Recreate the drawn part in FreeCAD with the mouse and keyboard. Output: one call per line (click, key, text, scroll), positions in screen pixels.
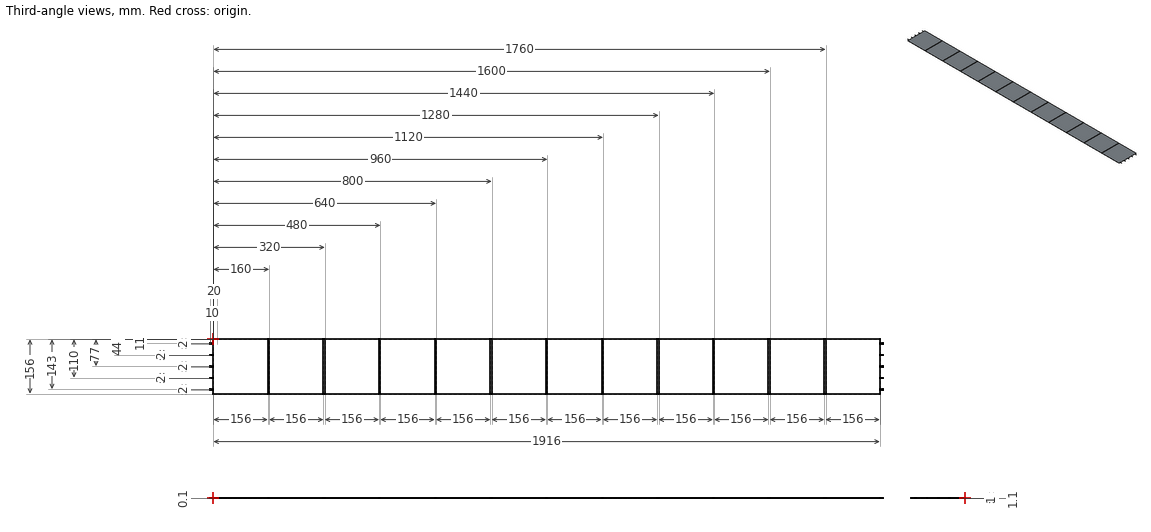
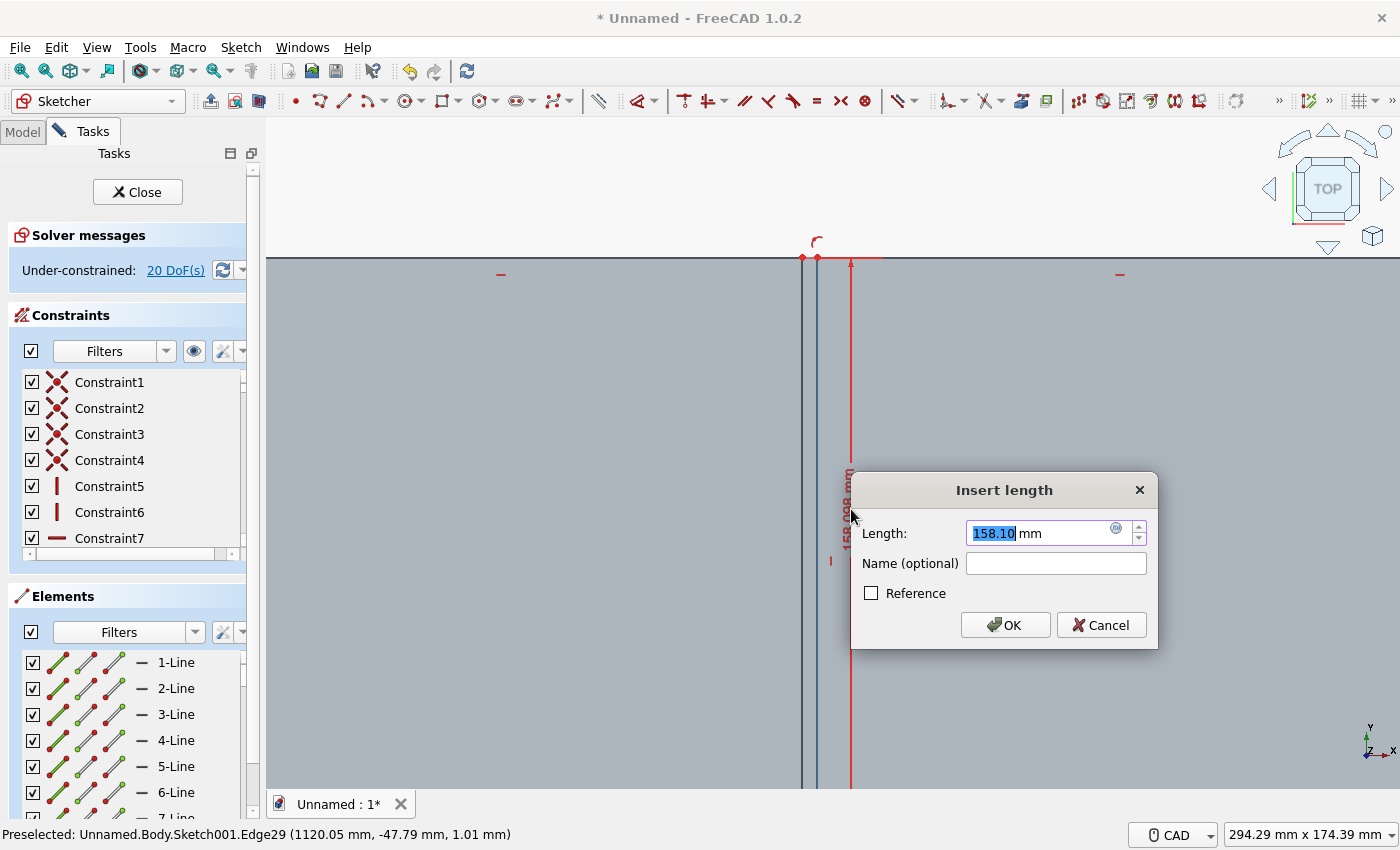
text(156)
key(Return)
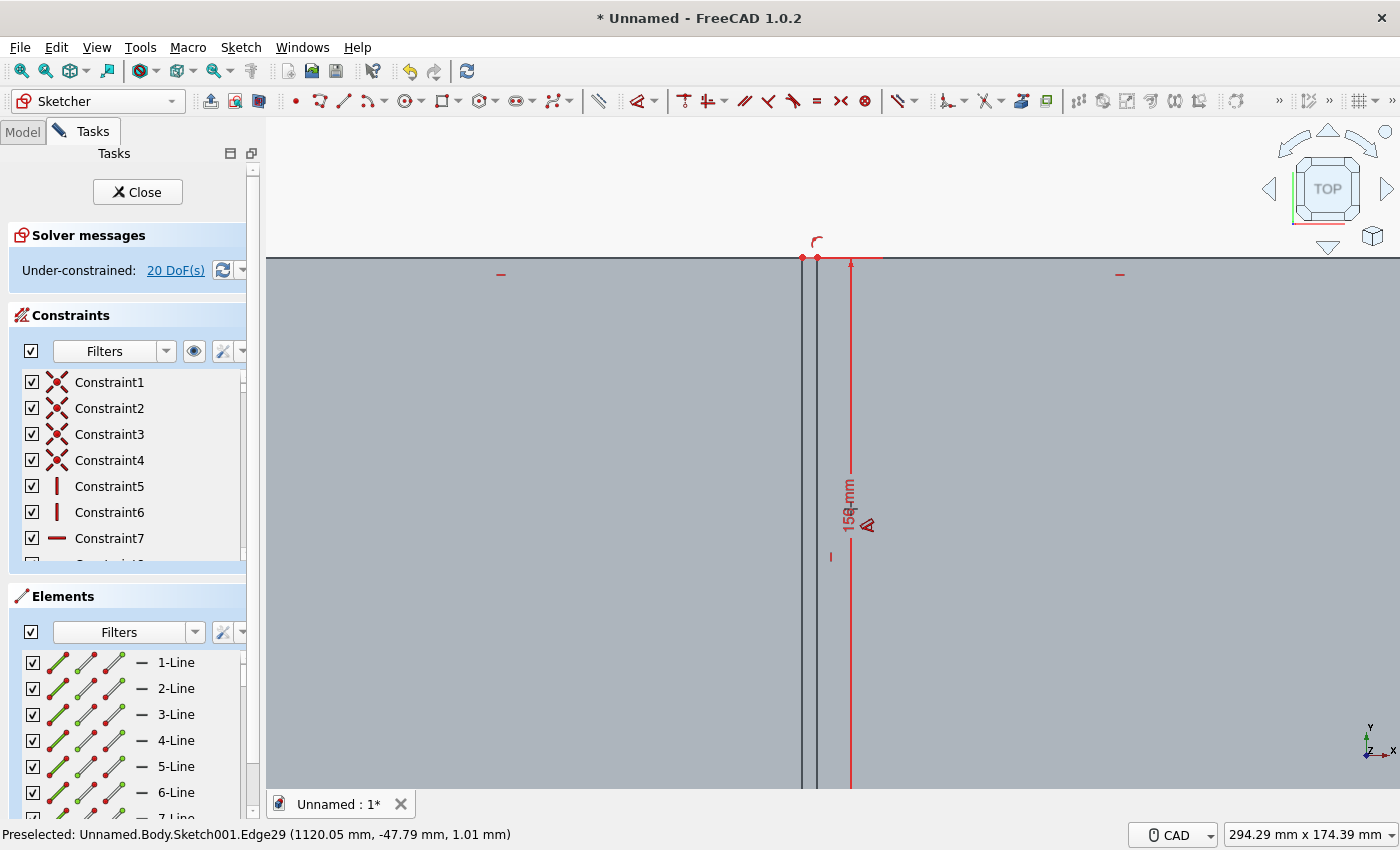
scroll(822, 442, down, 12)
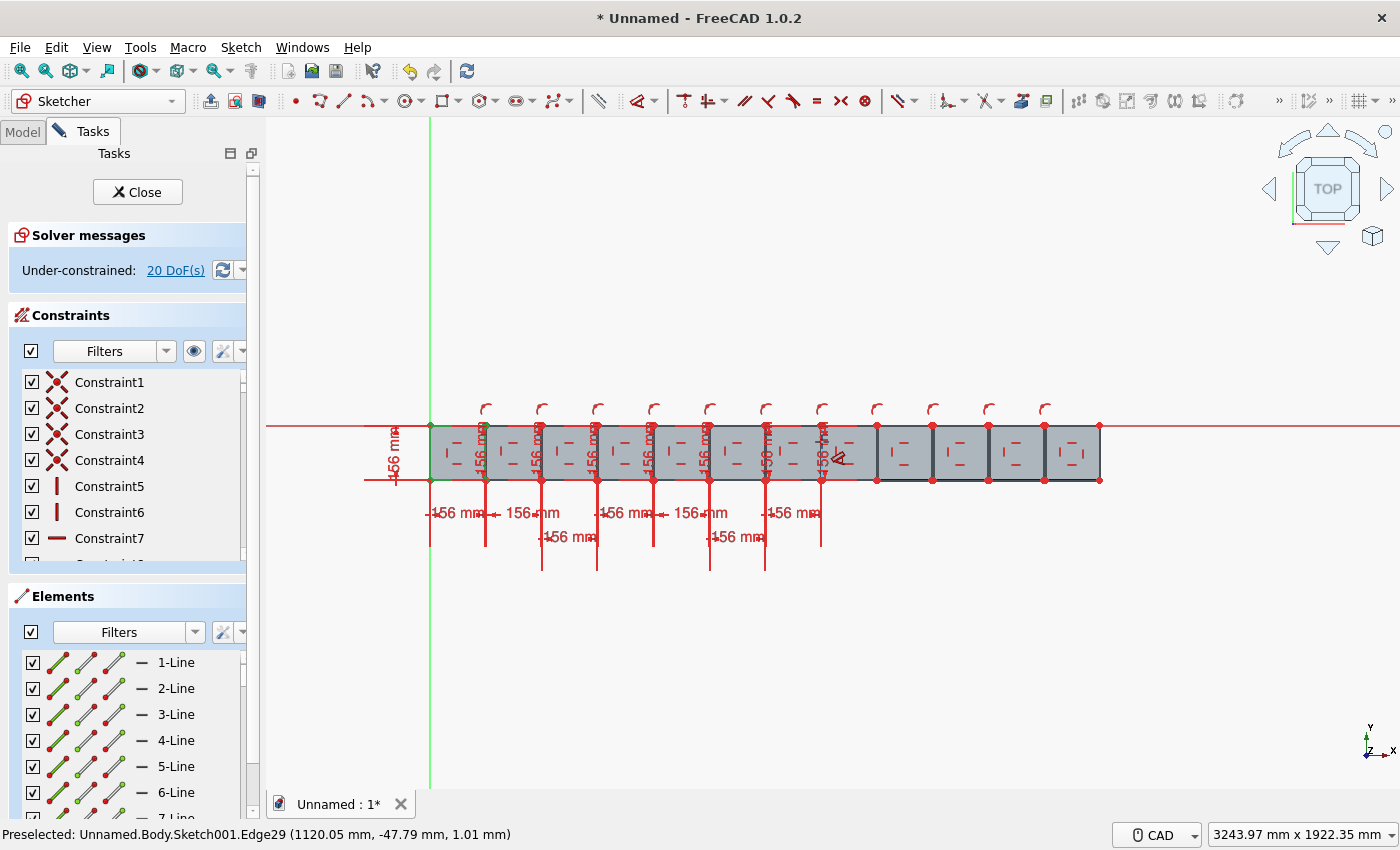
click(839, 480)
click(869, 514)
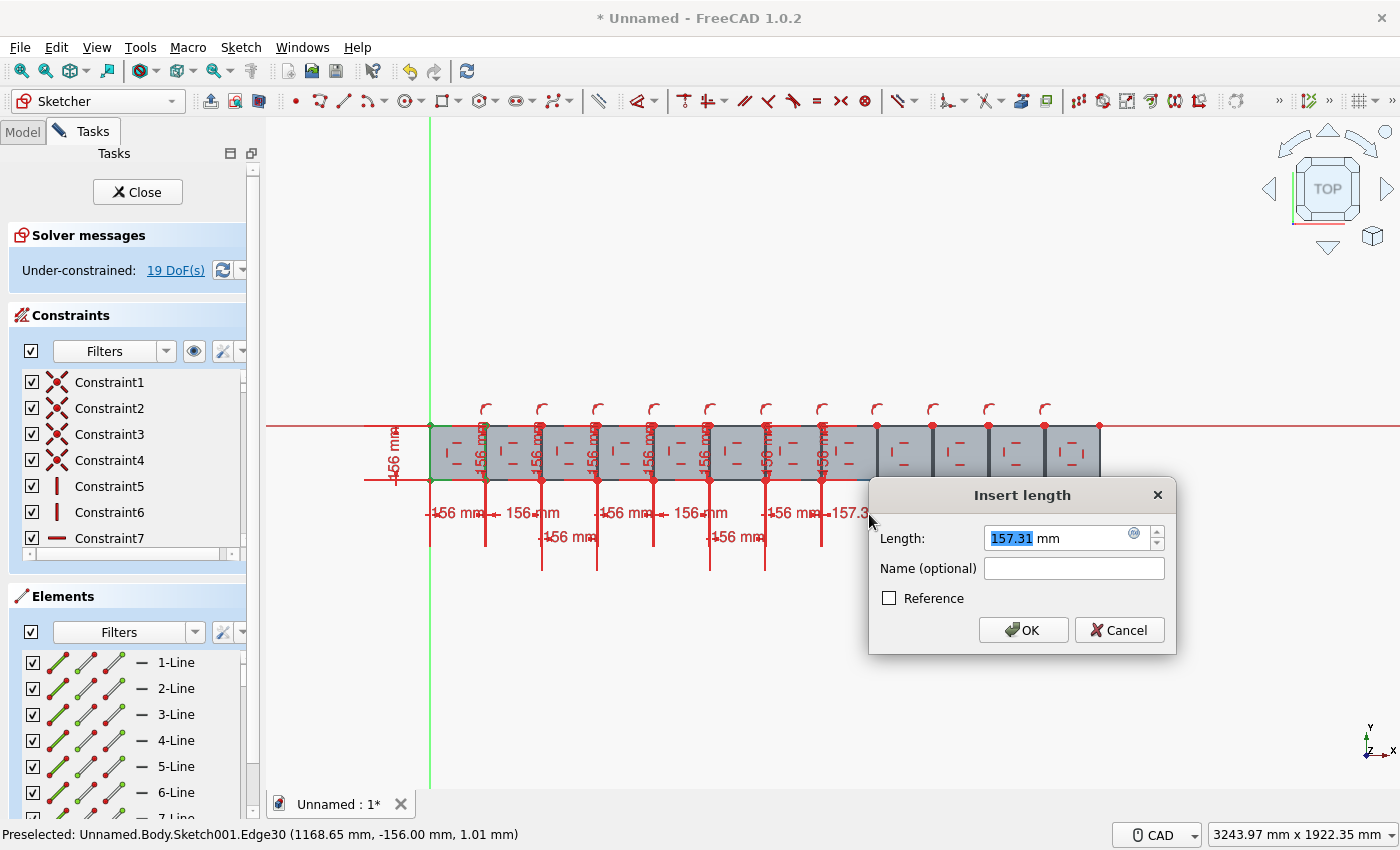
text(156)
key(Return)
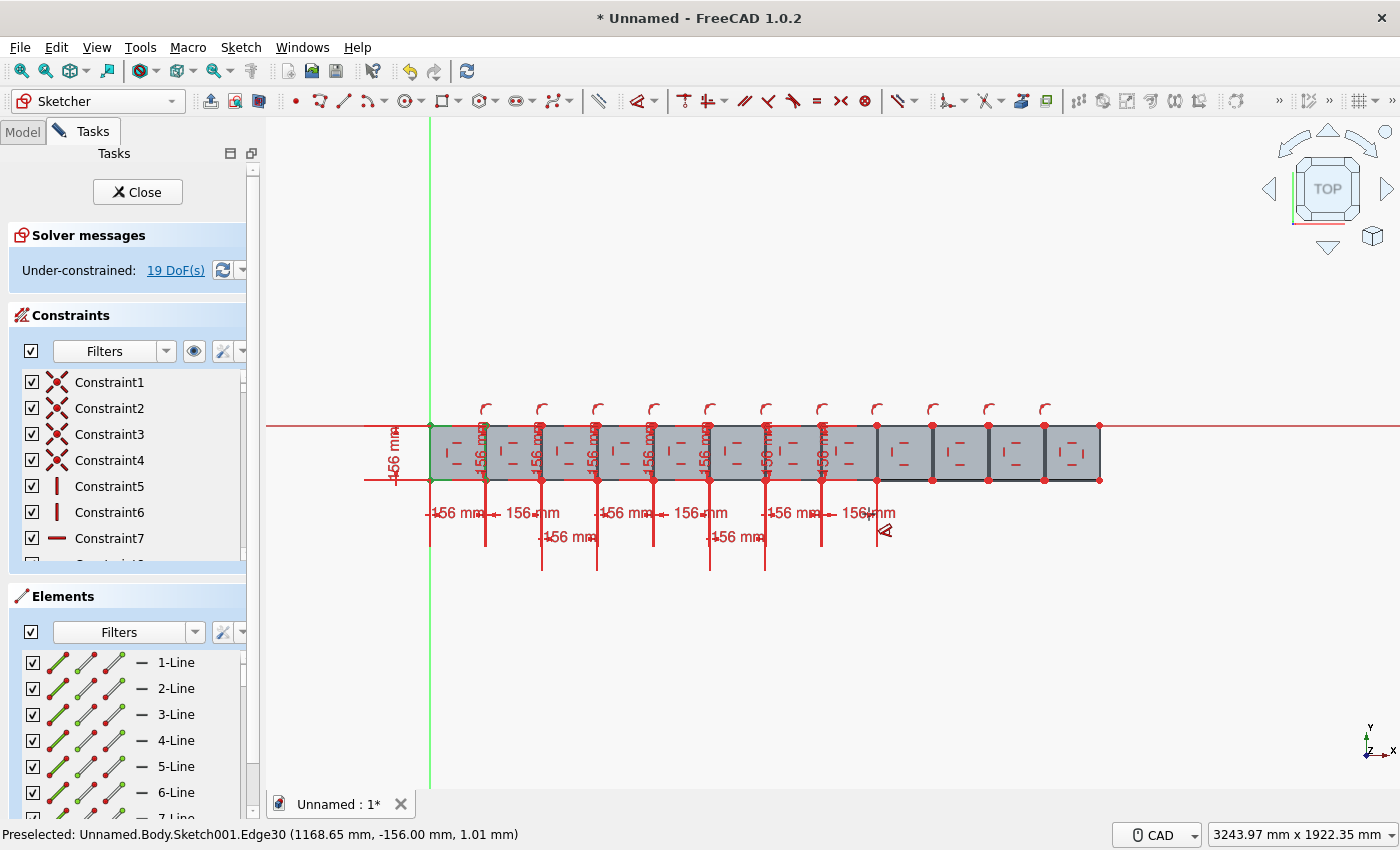
scroll(878, 442, up, 12)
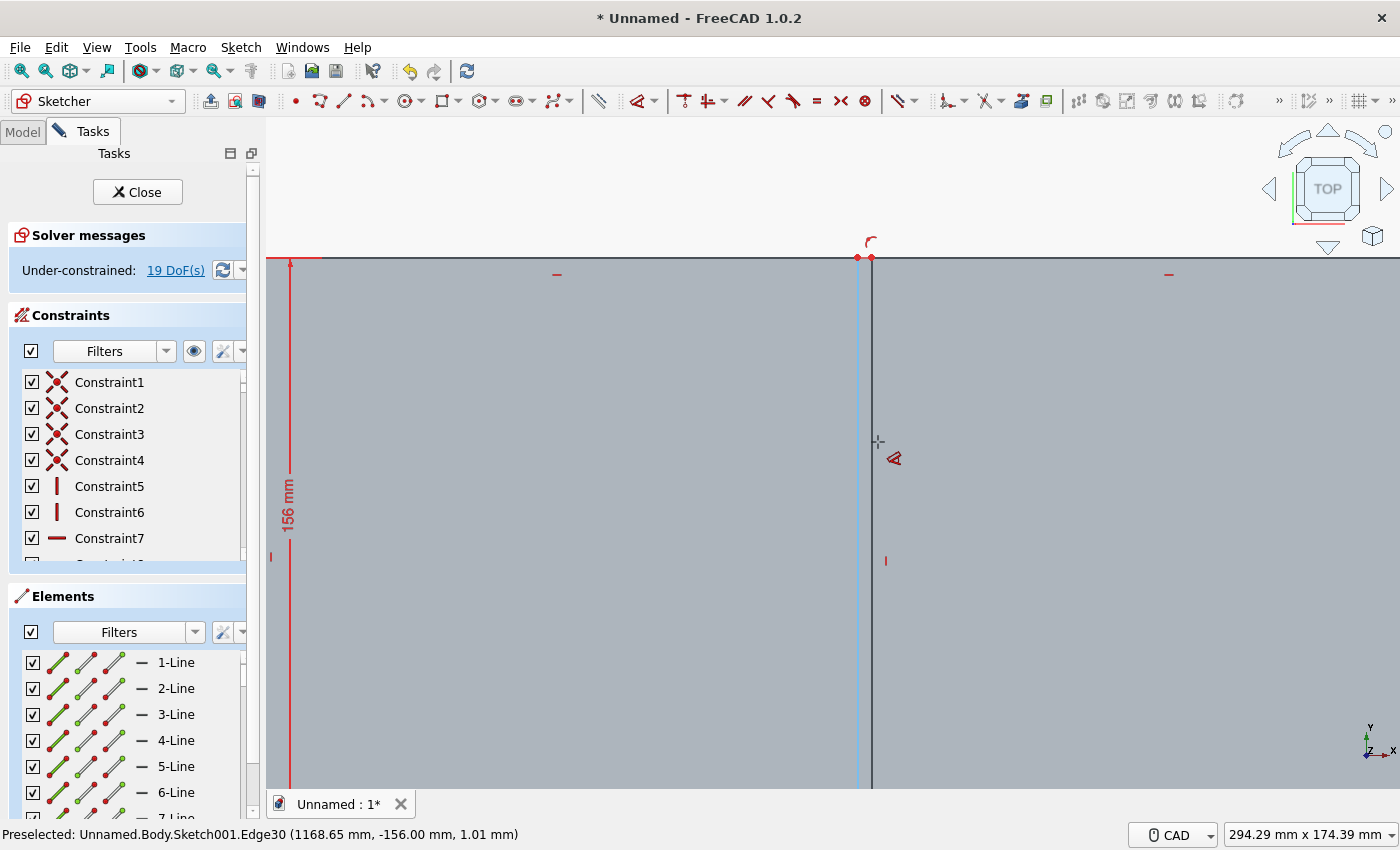
click(872, 441)
click(906, 509)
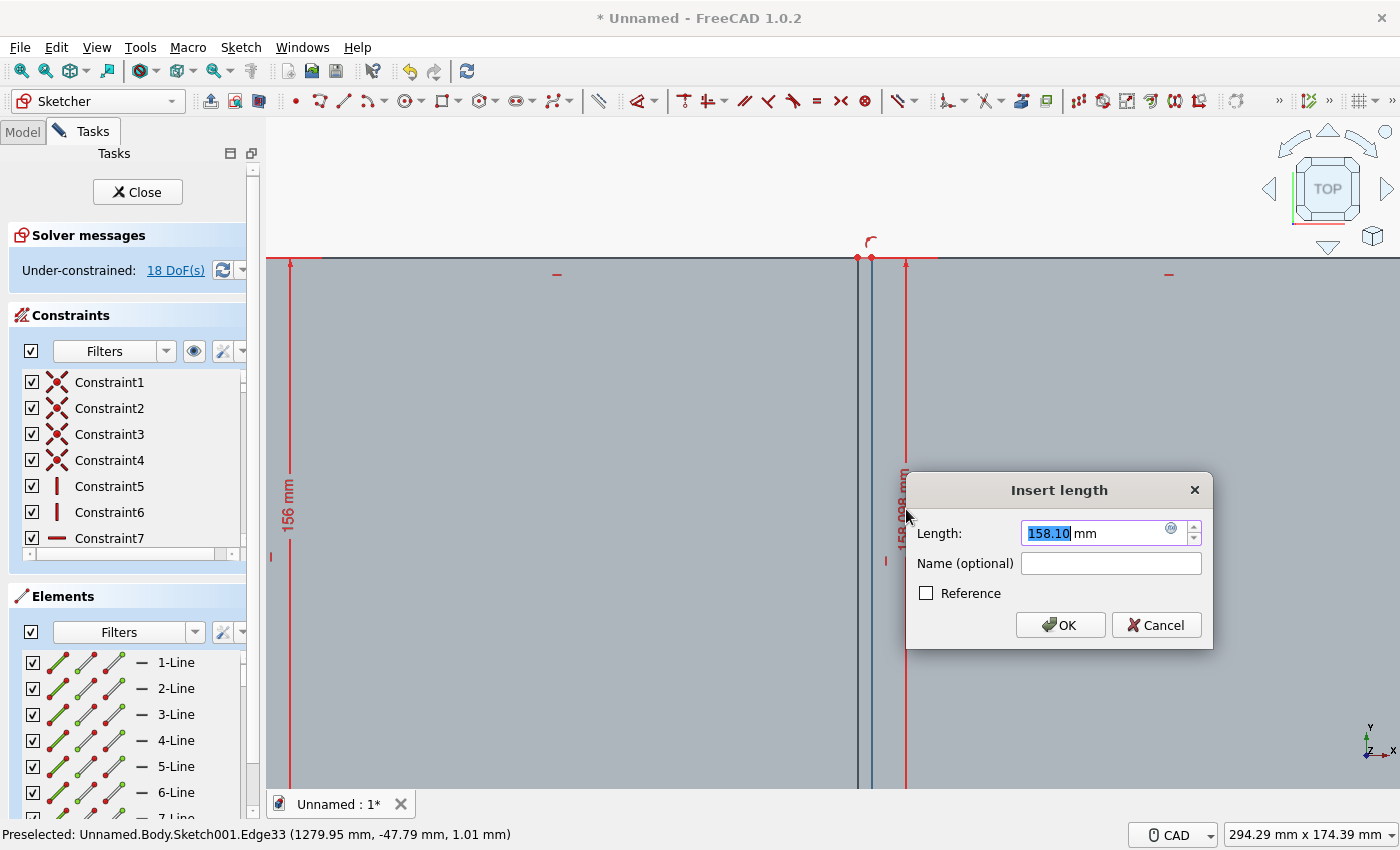
text(156)
key(Return)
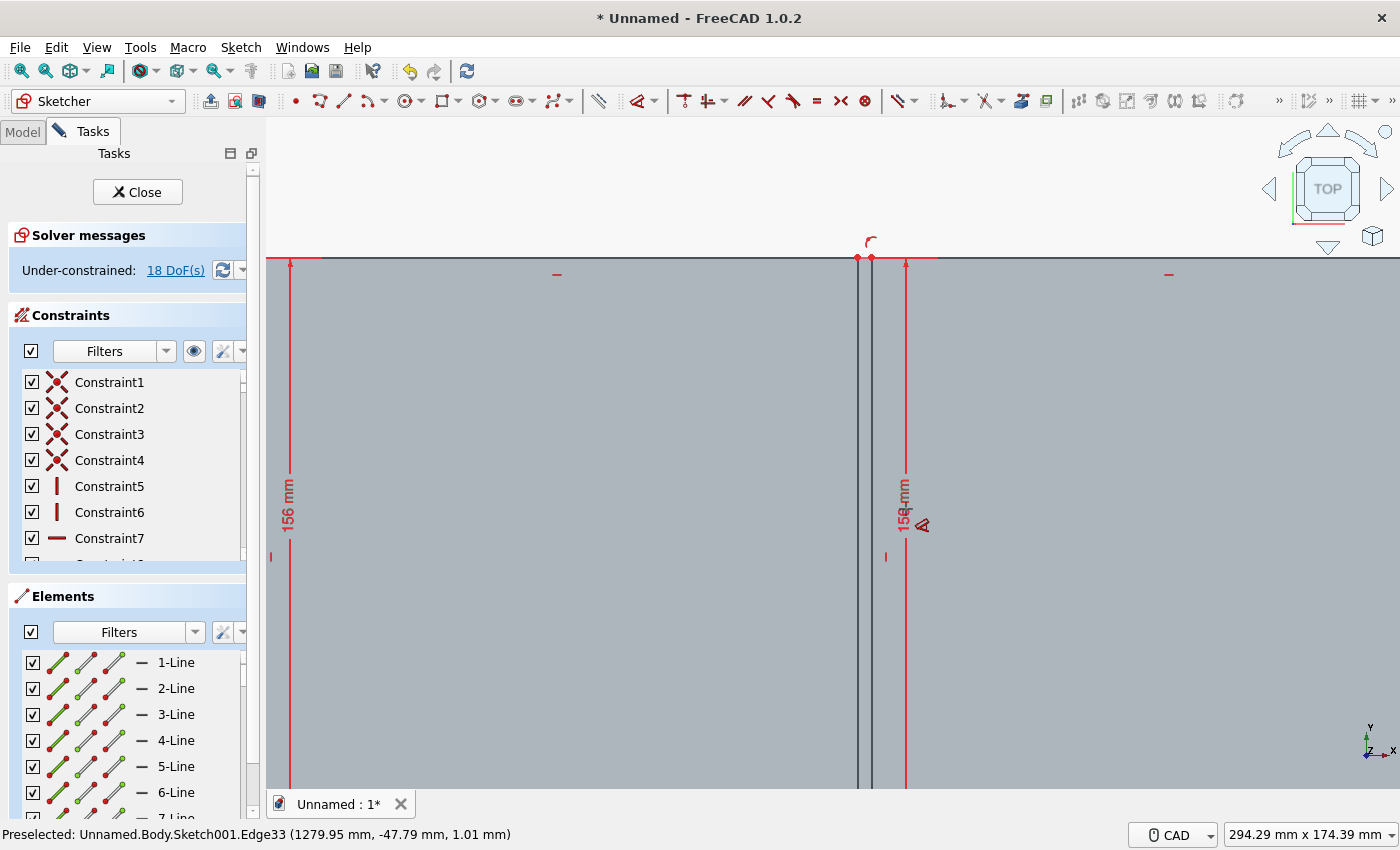
scroll(878, 442, down, 12)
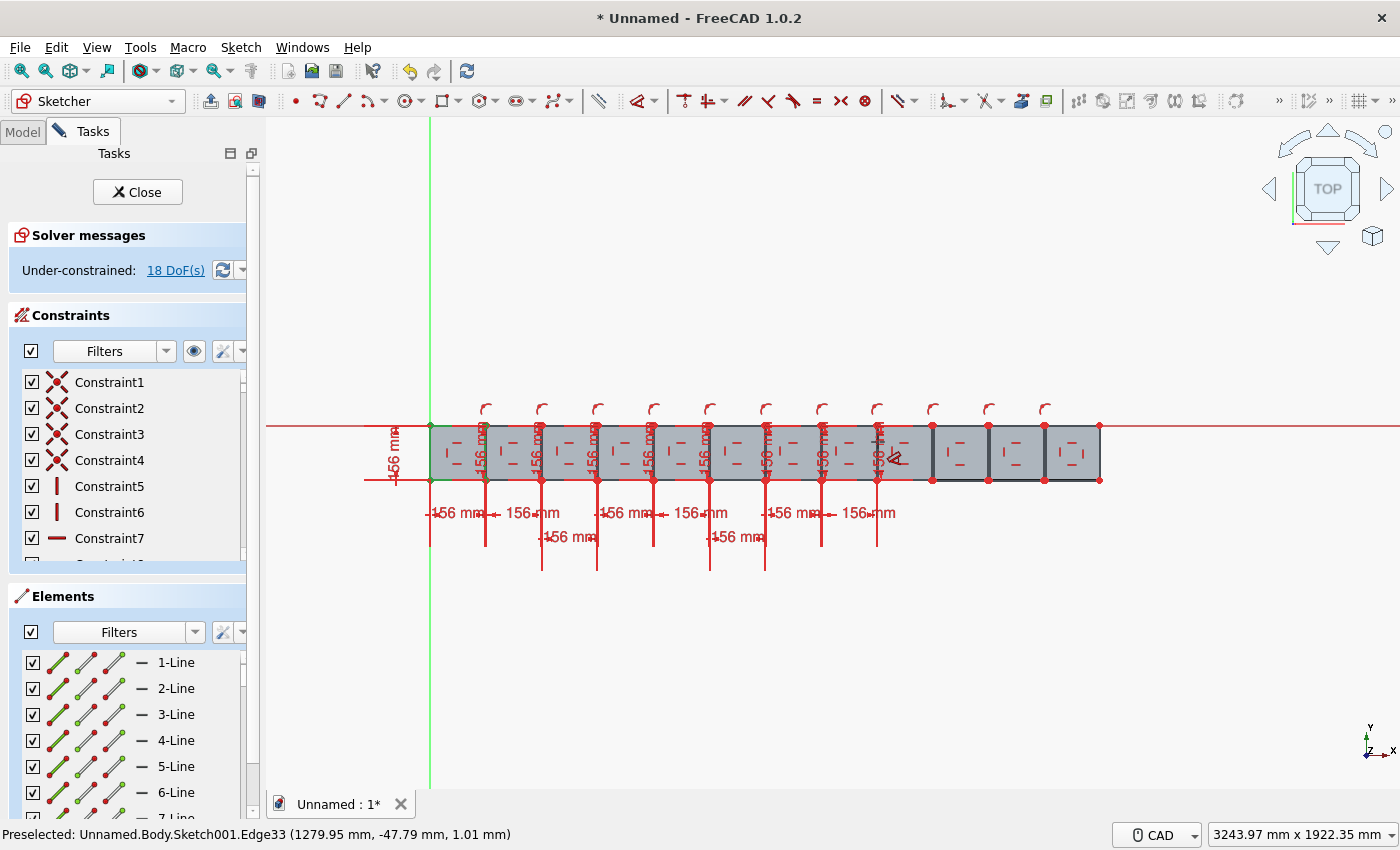
click(894, 480)
click(905, 538)